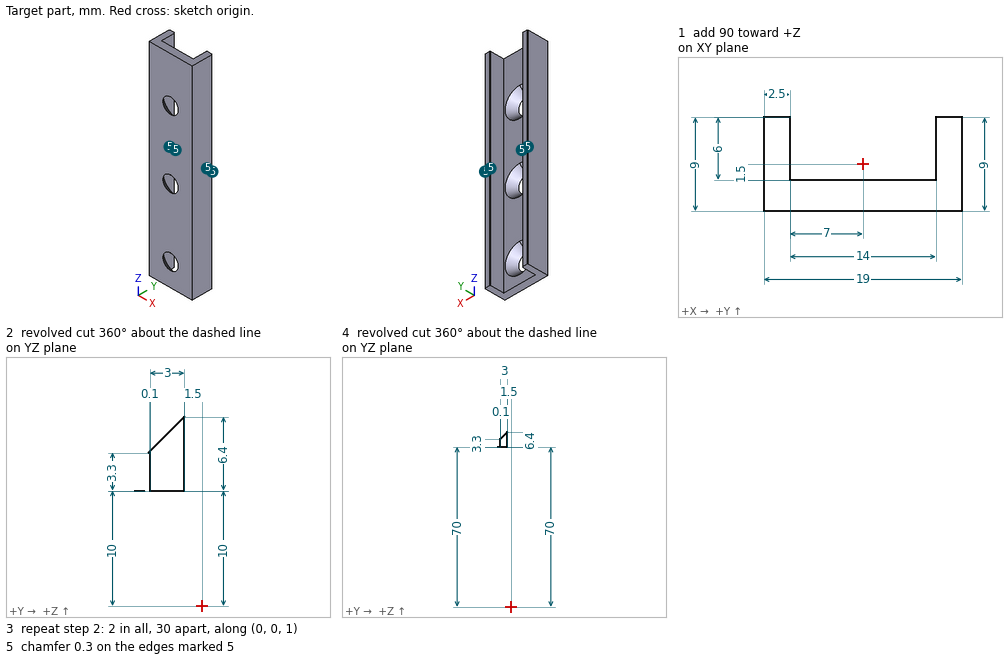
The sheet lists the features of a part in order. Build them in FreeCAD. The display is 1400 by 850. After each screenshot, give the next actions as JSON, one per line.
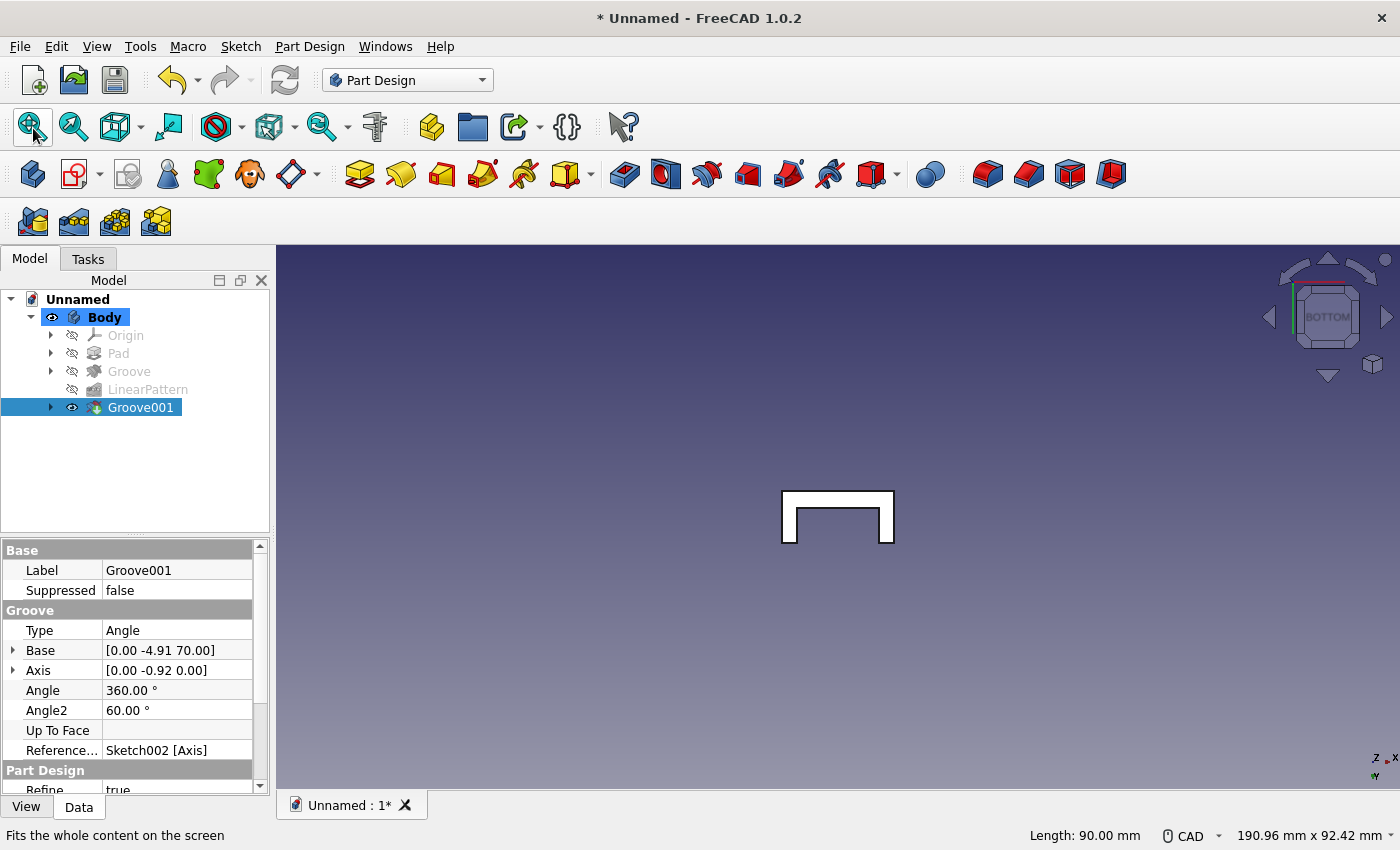
{"action": "key", "text": "4"}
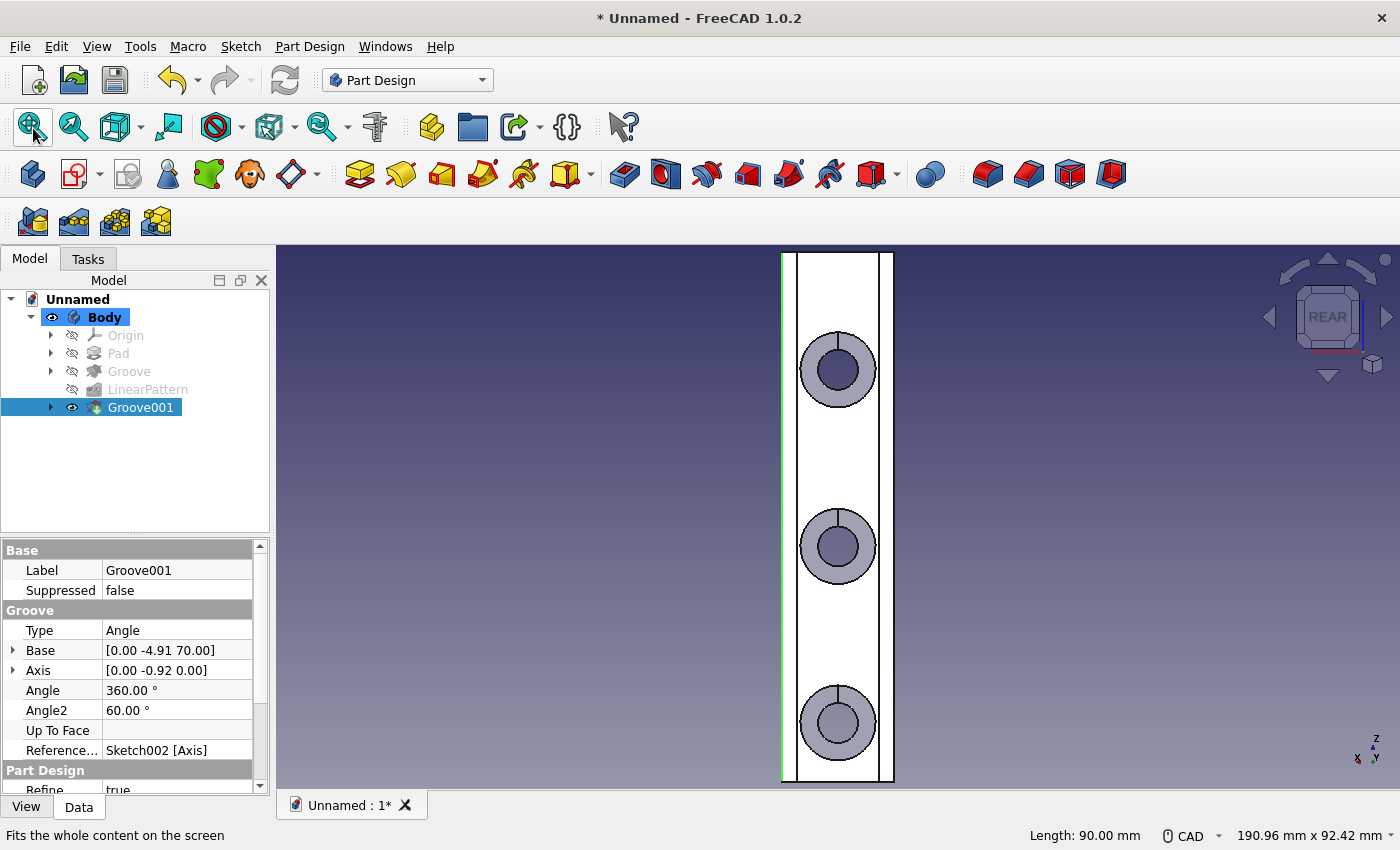
{"action": "left_click", "coordinate": [894, 516], "text": "ctrl"}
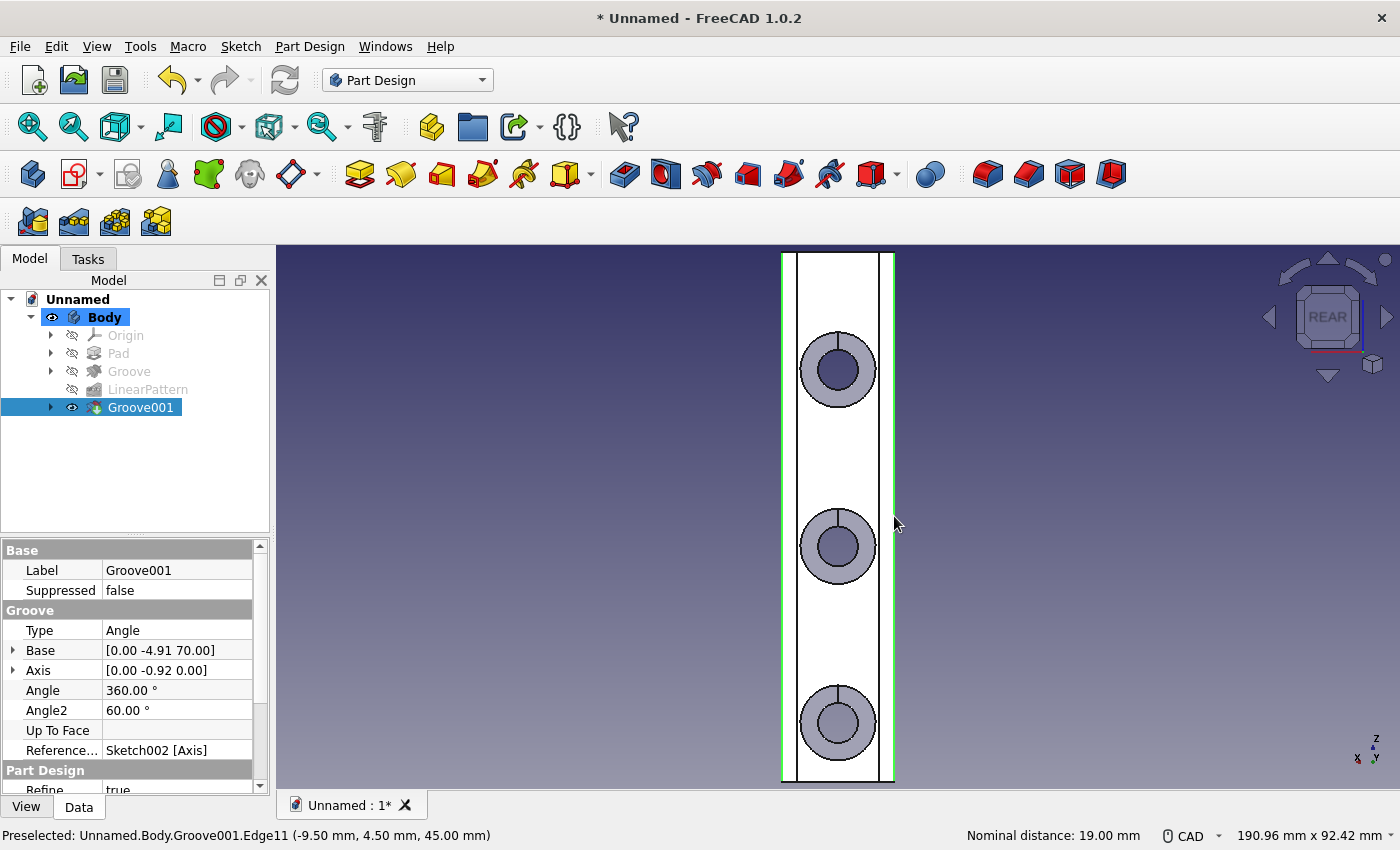
{"action": "left_click", "coordinate": [879, 516], "text": "ctrl"}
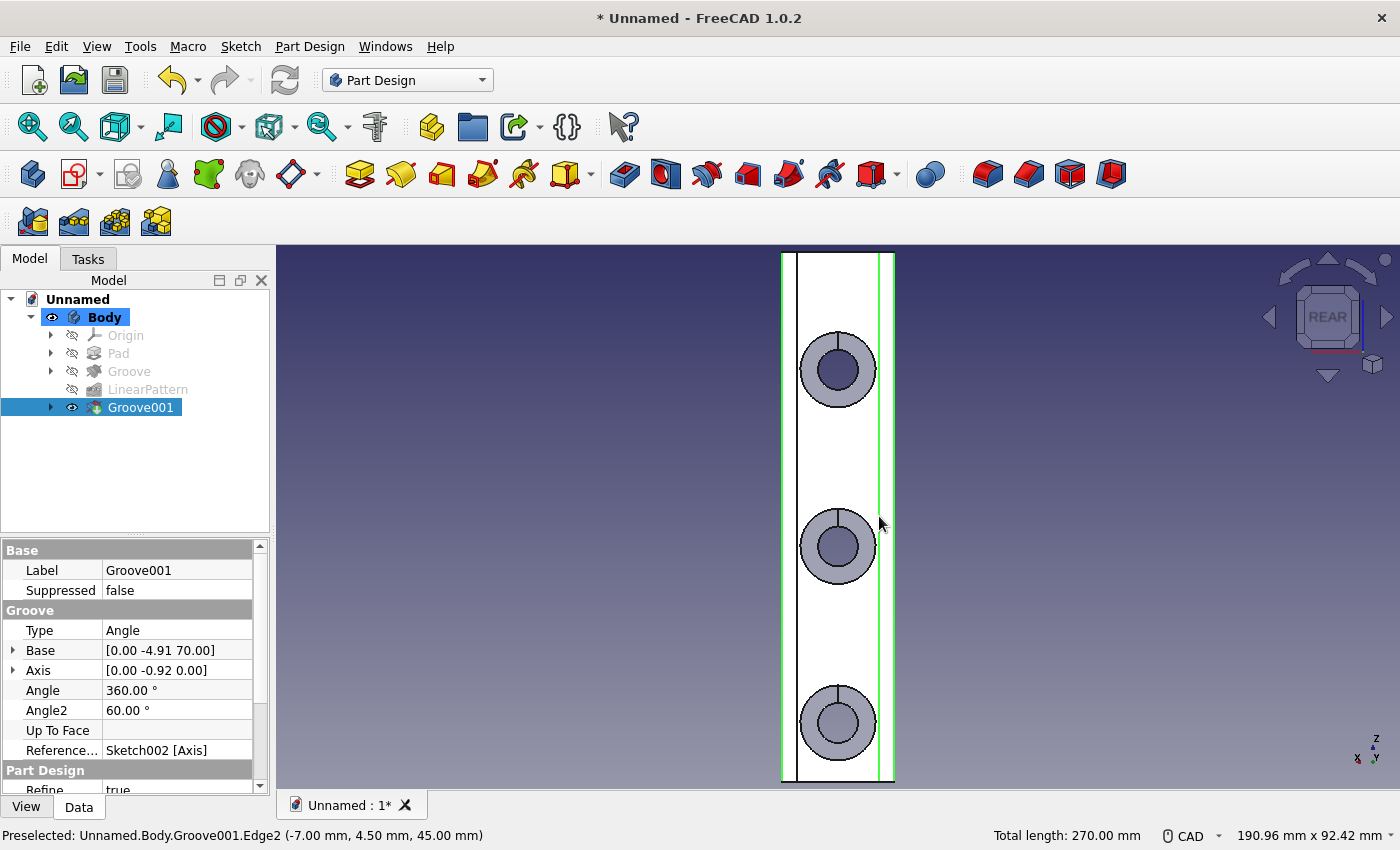
{"action": "left_click", "coordinate": [797, 516], "text": "ctrl"}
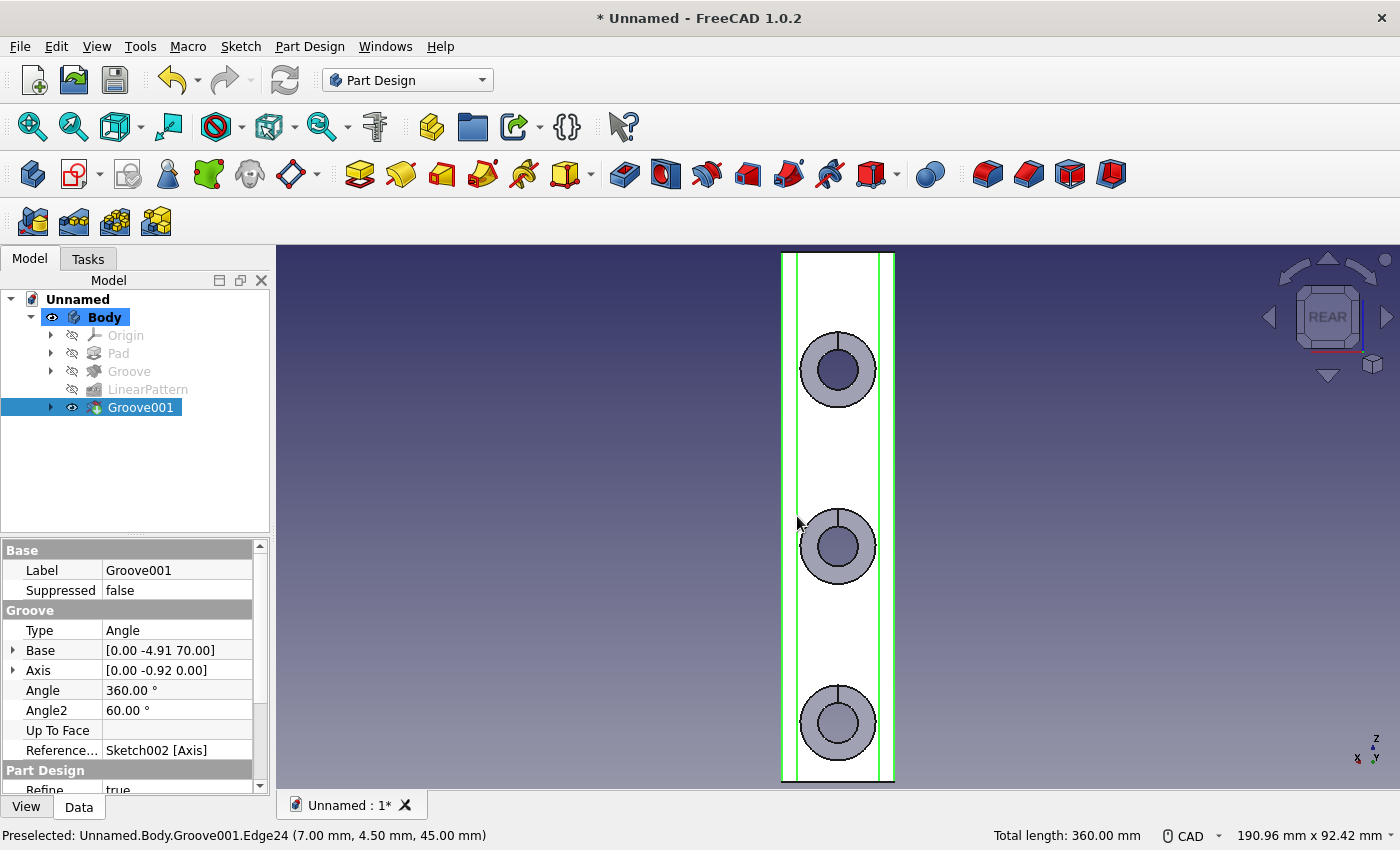
{"action": "left_click", "coordinate": [1029, 174]}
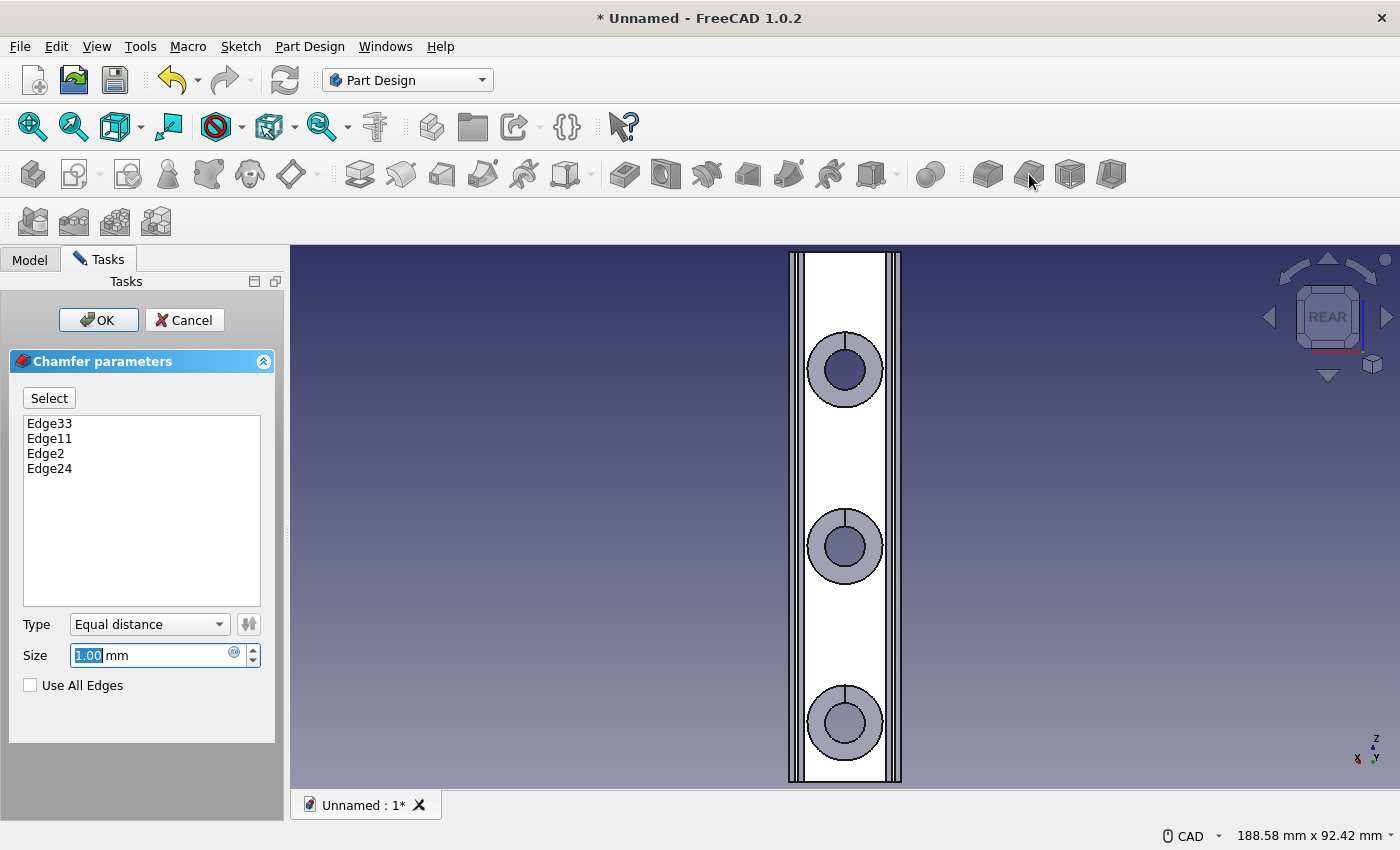
{"action": "type", "text": "0.3"}
{"action": "key", "text": "Tab"}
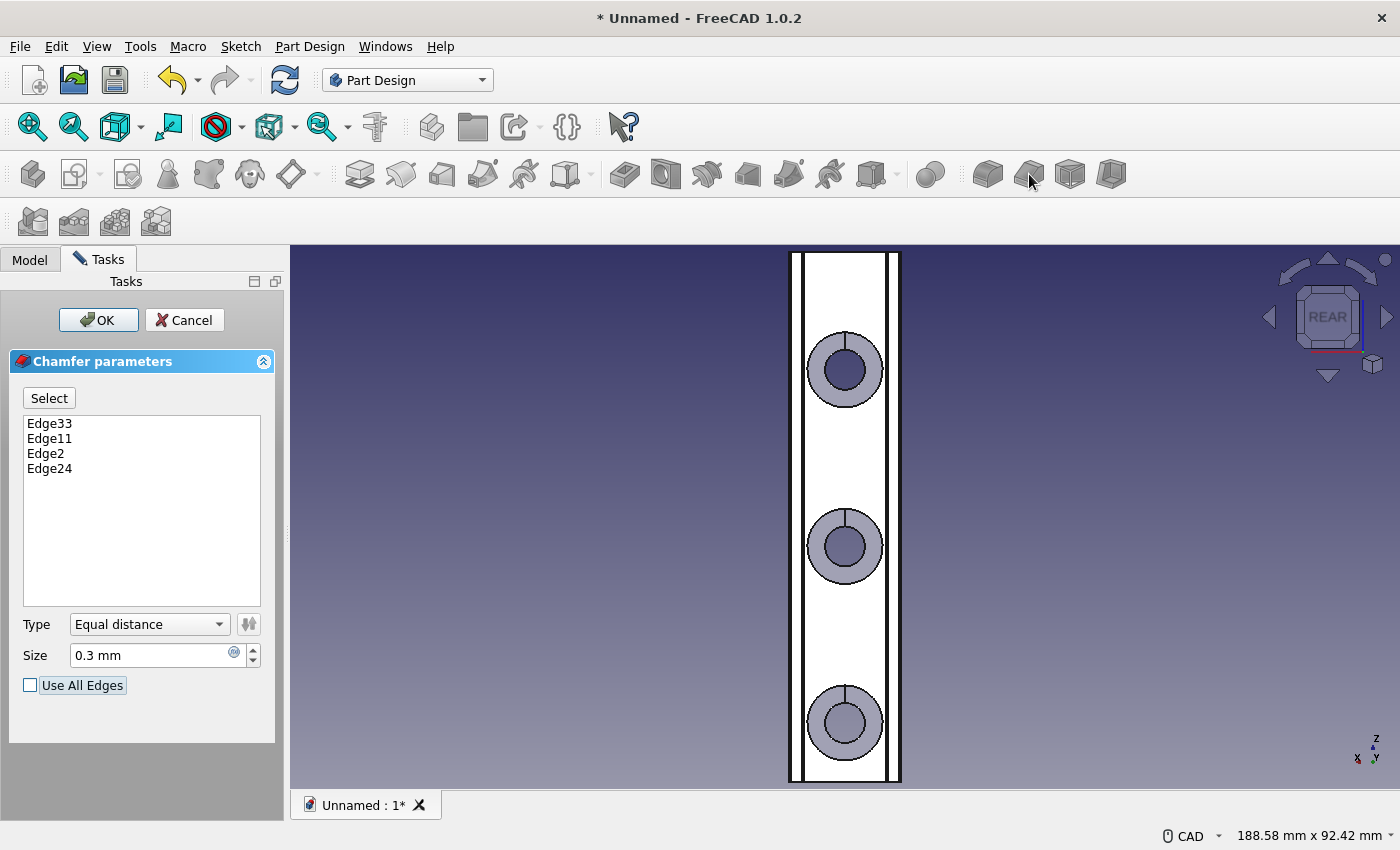
{"action": "left_click", "coordinate": [99, 320]}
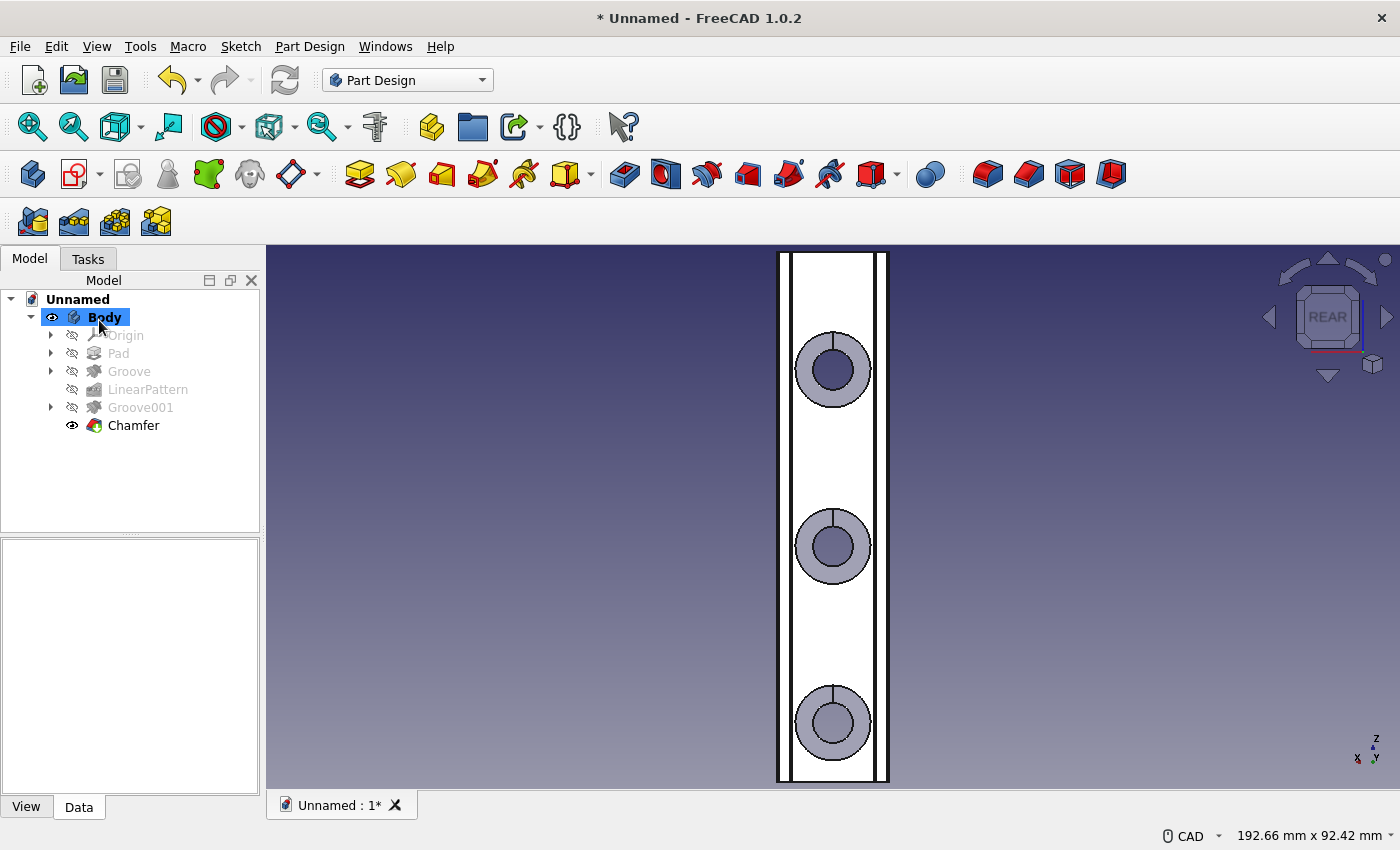
{"action": "key", "text": "0"}